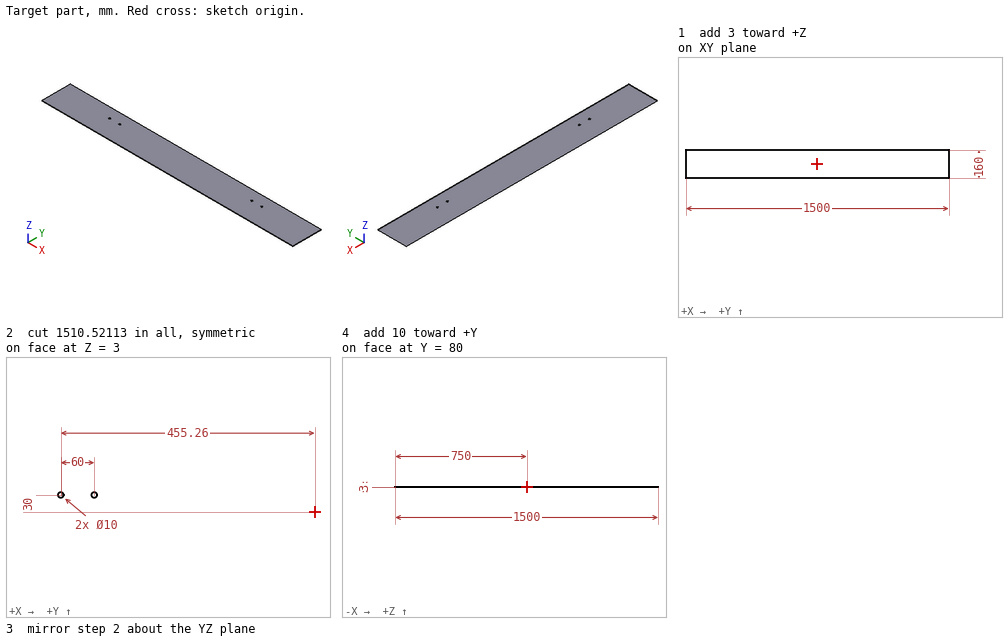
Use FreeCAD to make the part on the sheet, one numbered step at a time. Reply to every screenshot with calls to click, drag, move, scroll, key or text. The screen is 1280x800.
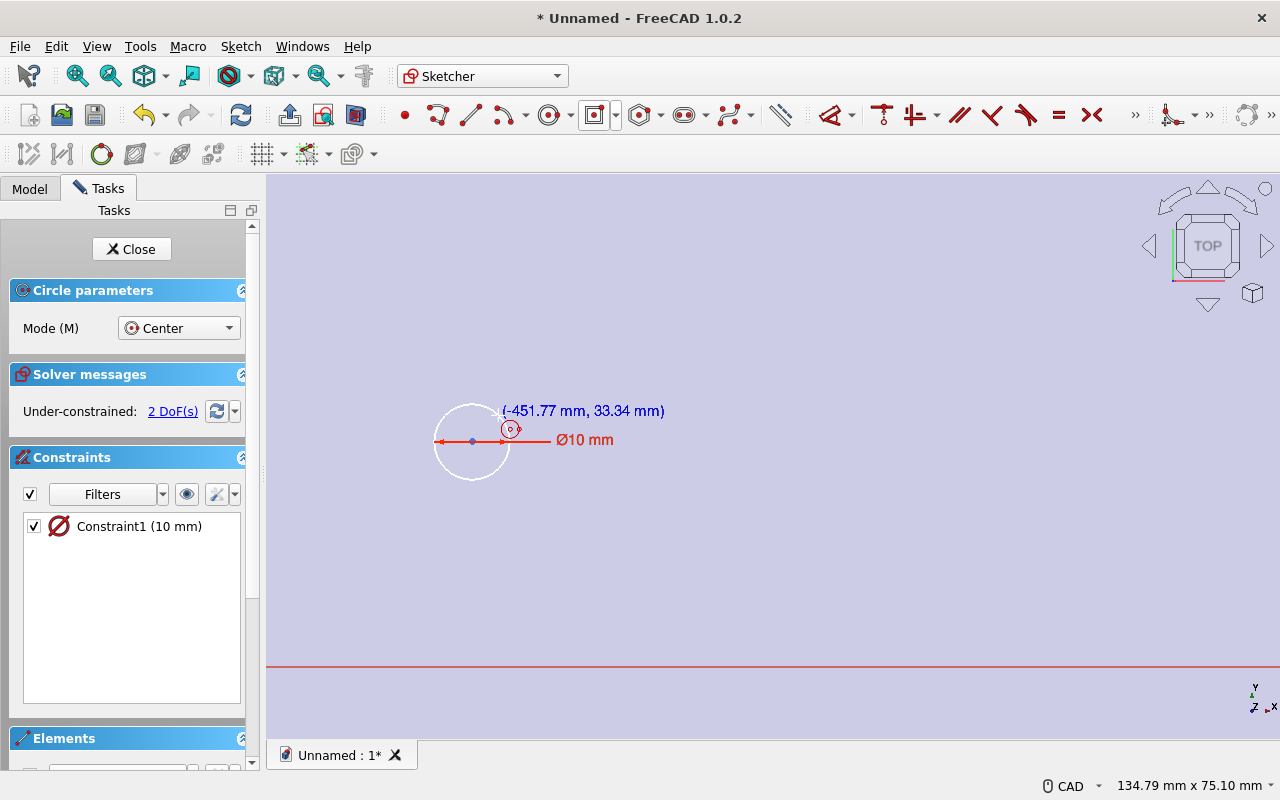
click(923, 441)
move(950, 415)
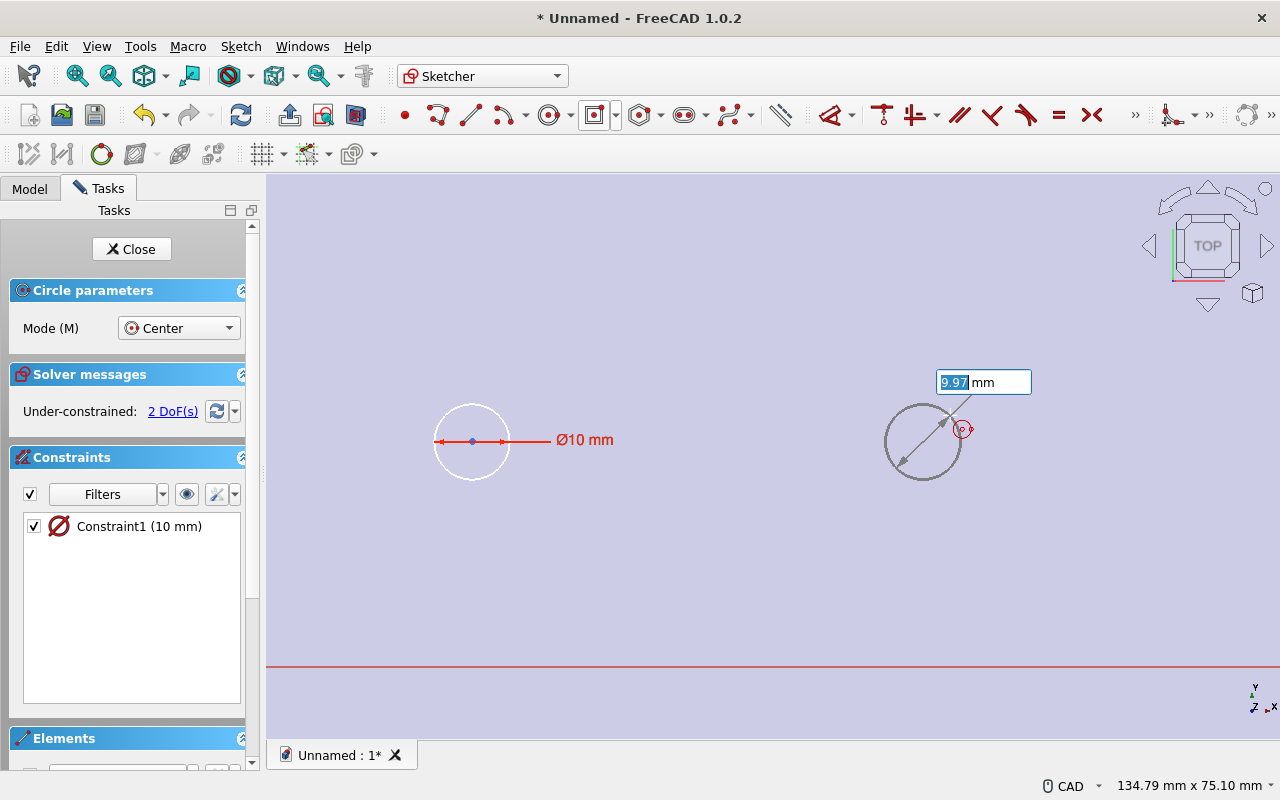
text(10)
key(Return)
key(Escape)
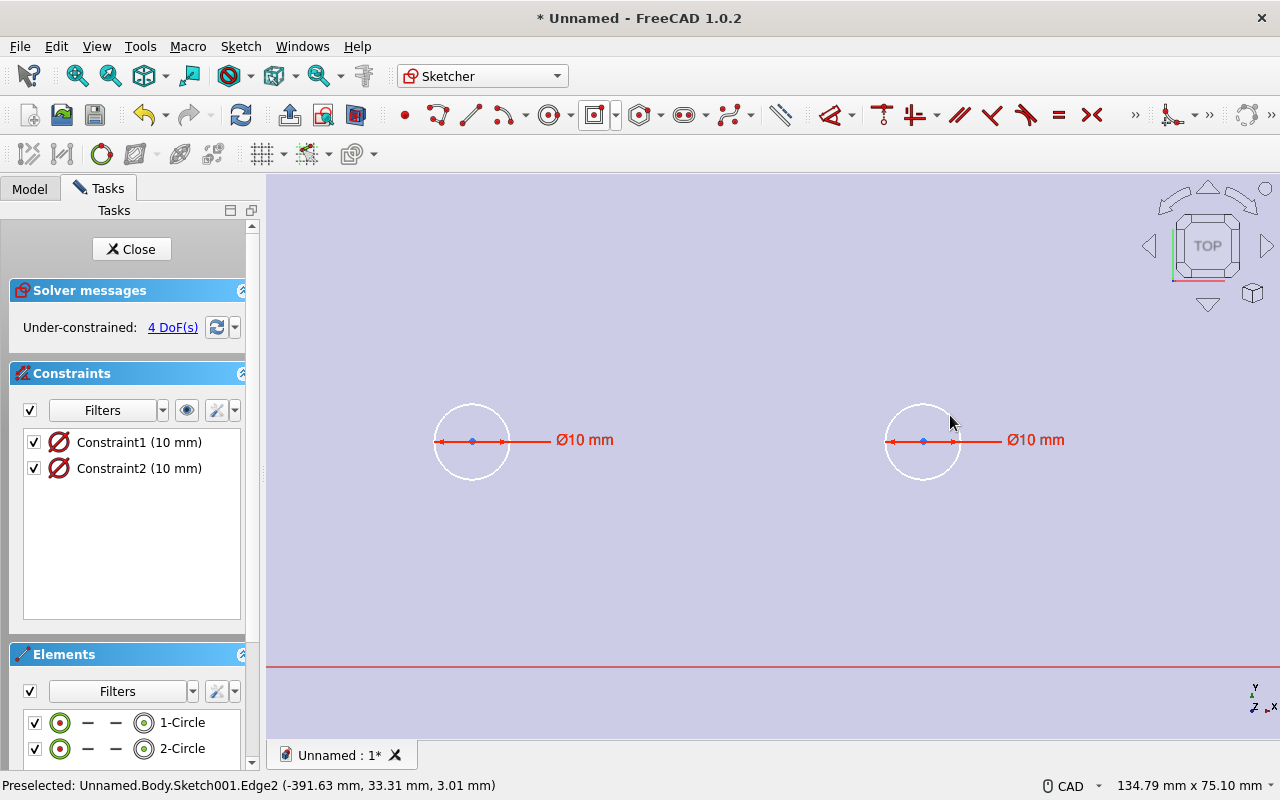
click(472, 442)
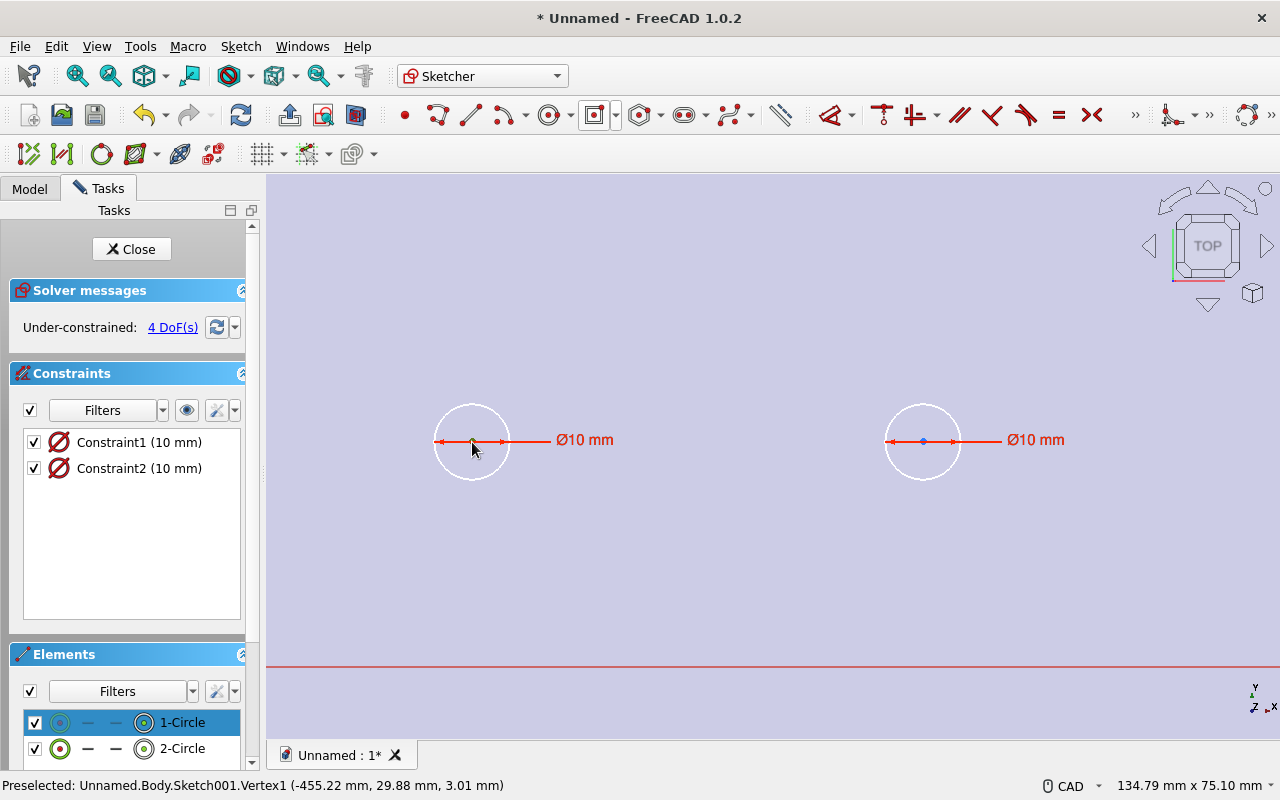
click(923, 442)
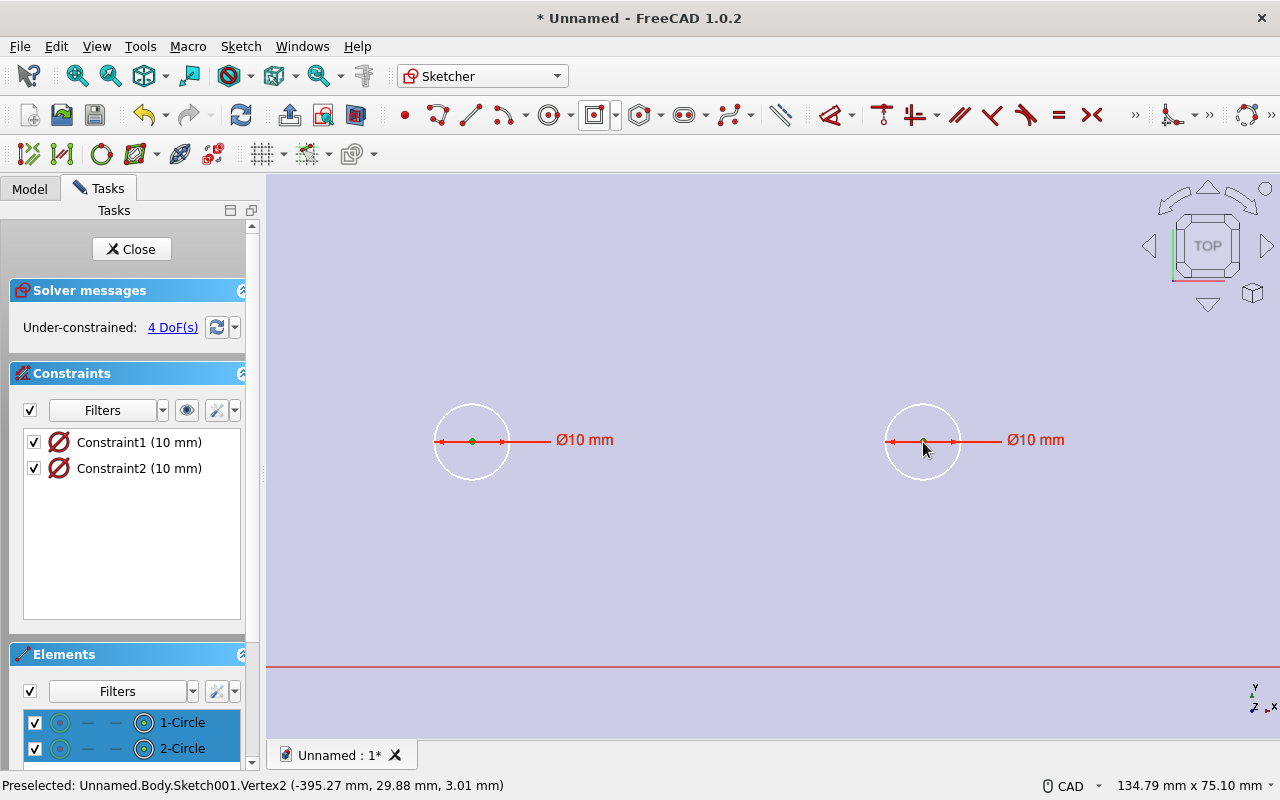
key(h)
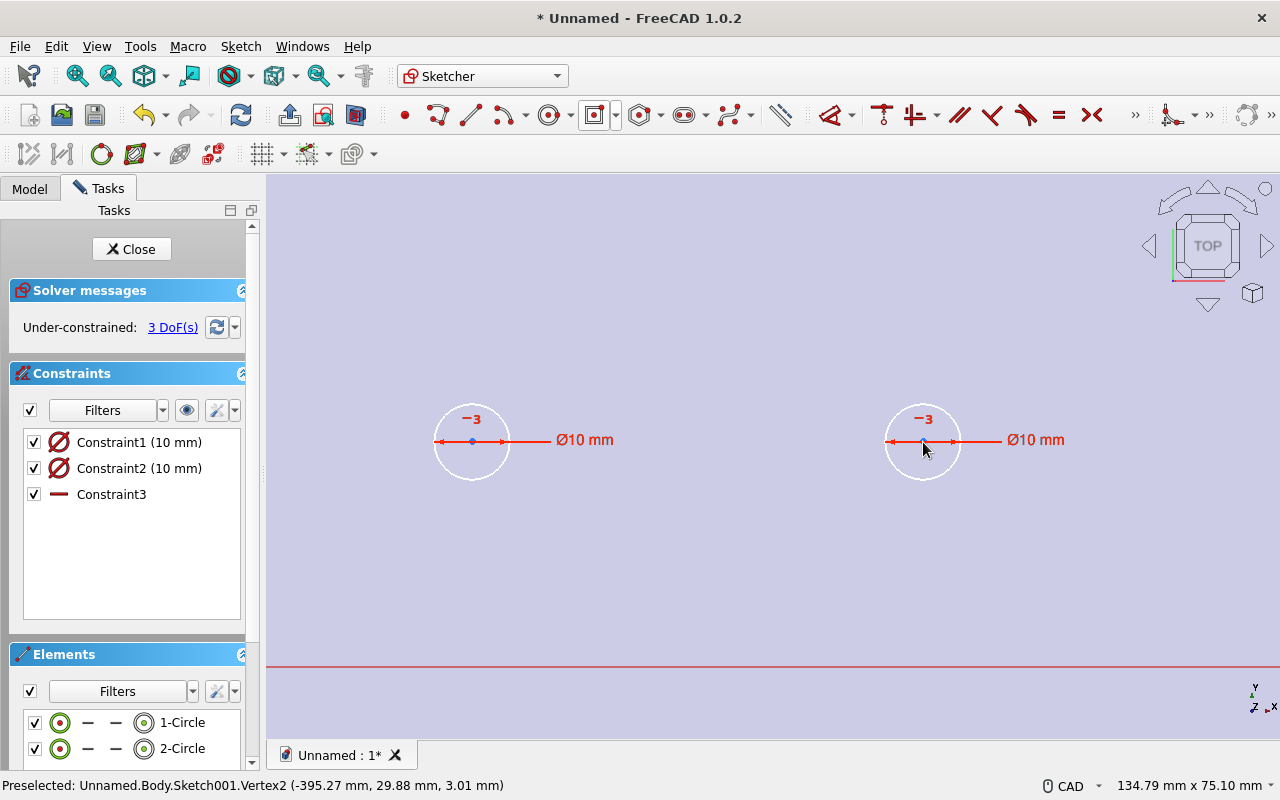
click(472, 442)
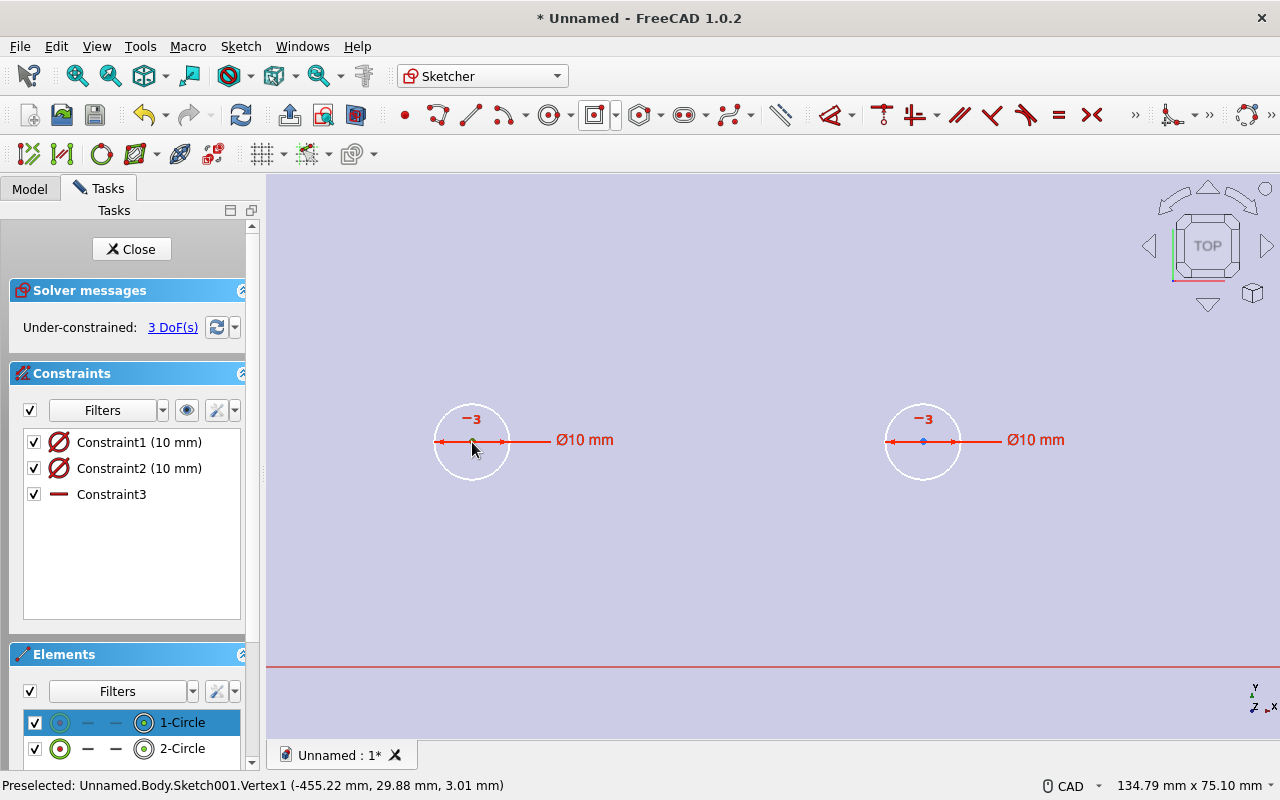
click(852, 116)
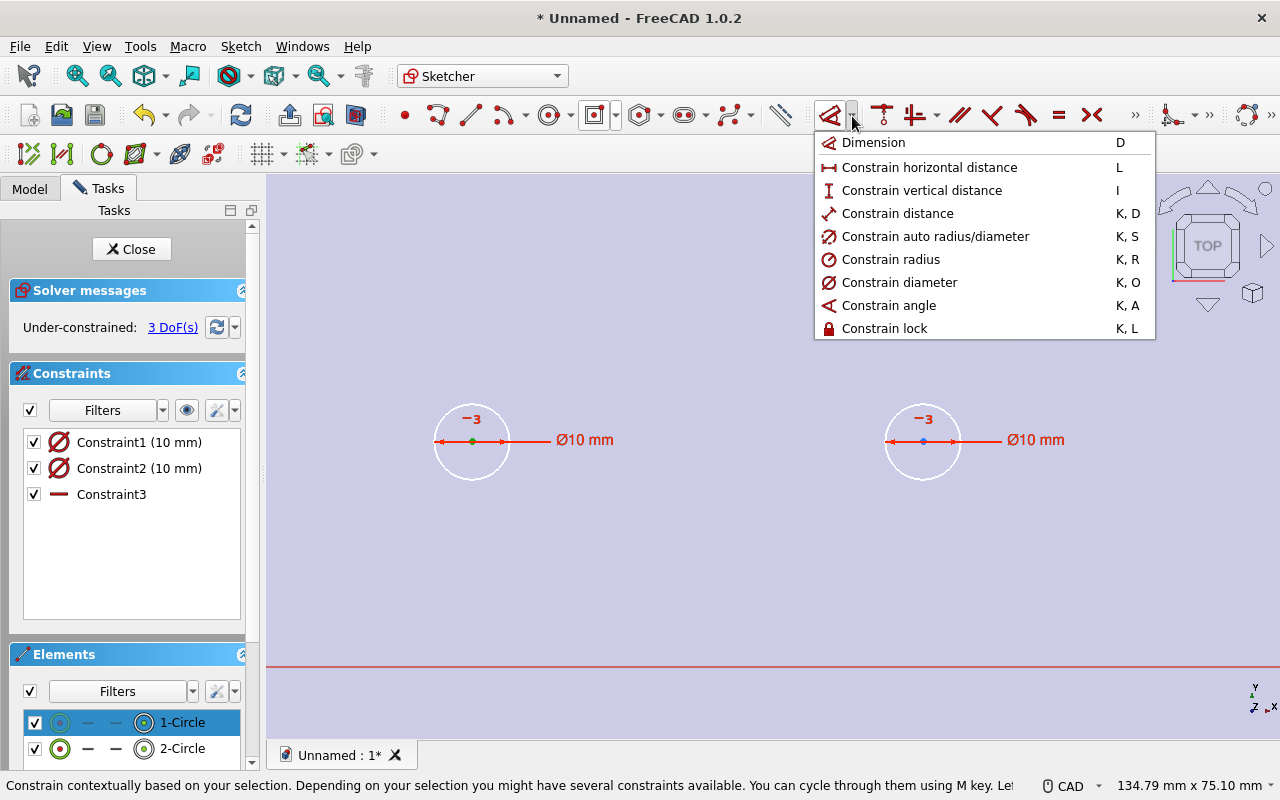
click(985, 190)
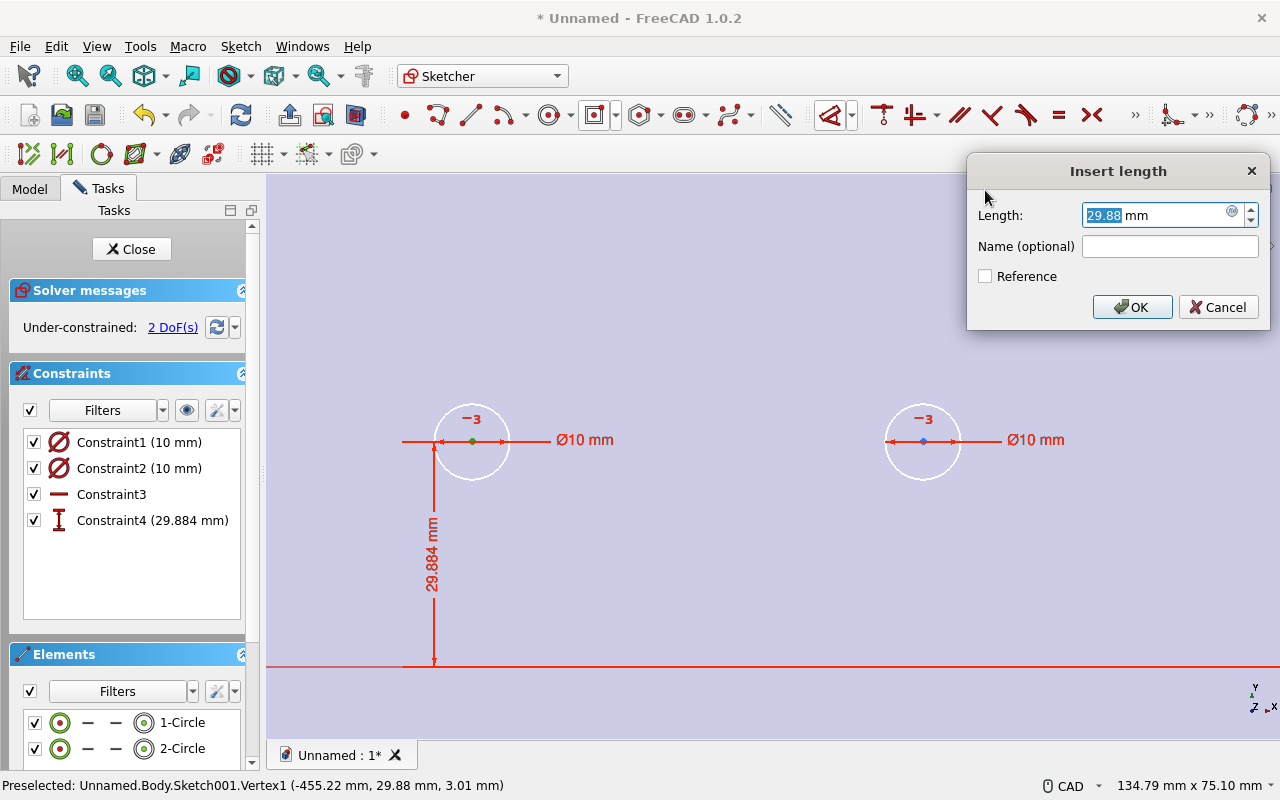
text(30)
key(Return)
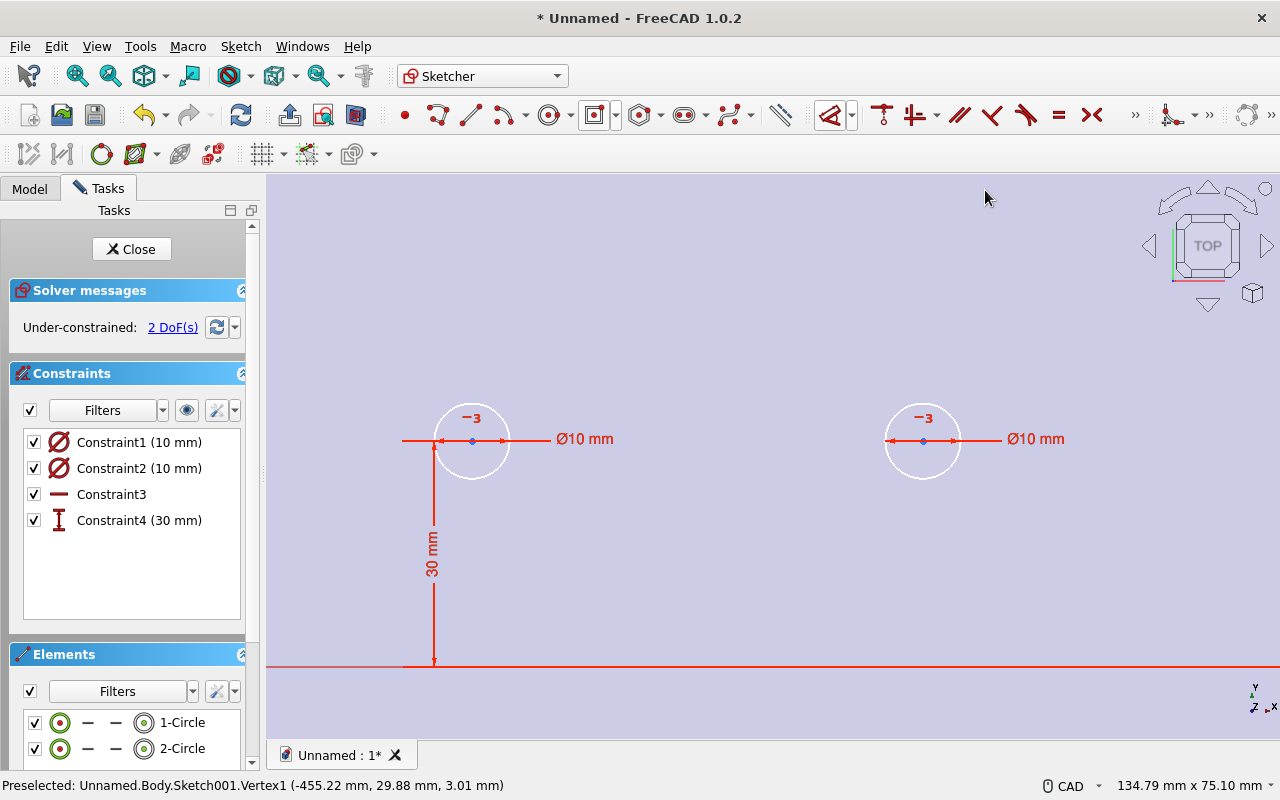
click(472, 441)